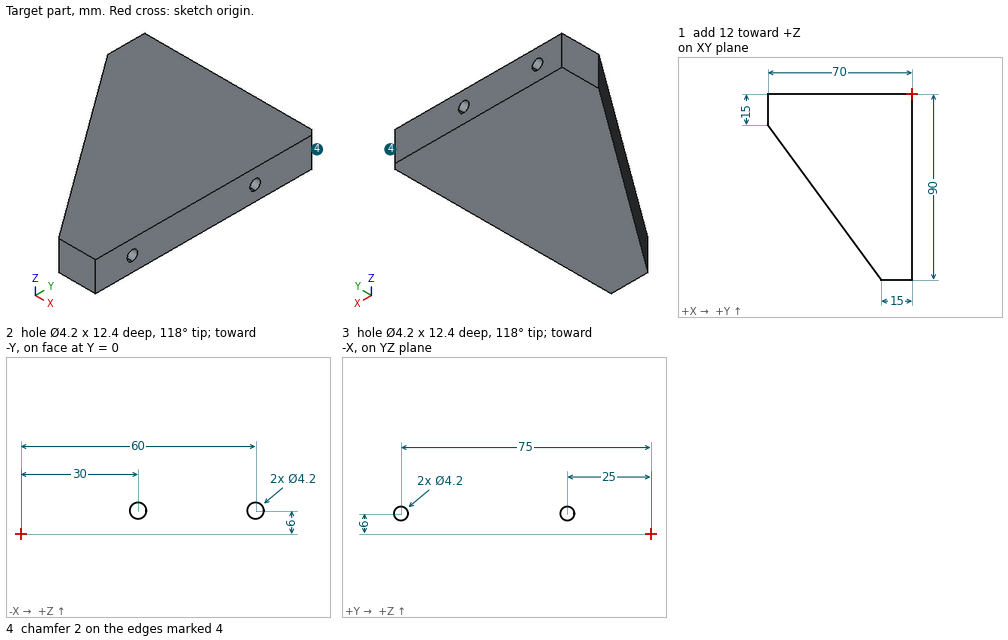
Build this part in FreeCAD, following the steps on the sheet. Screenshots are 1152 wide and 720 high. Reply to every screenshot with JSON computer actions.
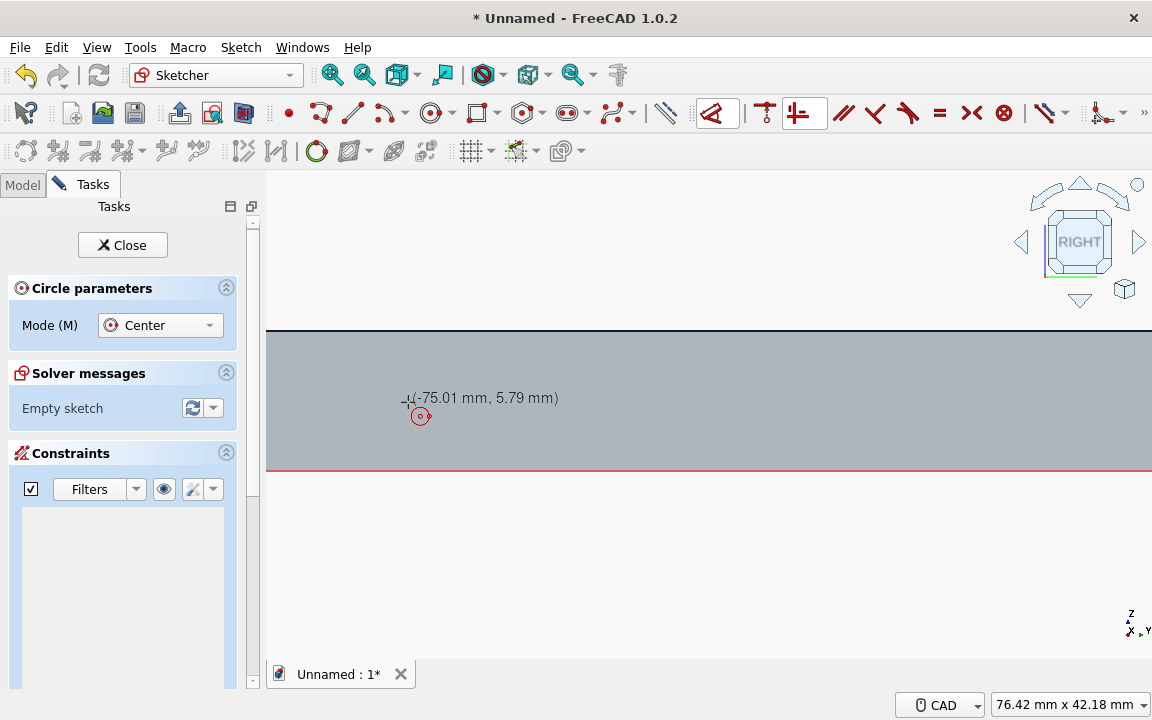
{"action": "left_click", "coordinate": [408, 401]}
{"action": "left_click", "coordinate": [425, 384]}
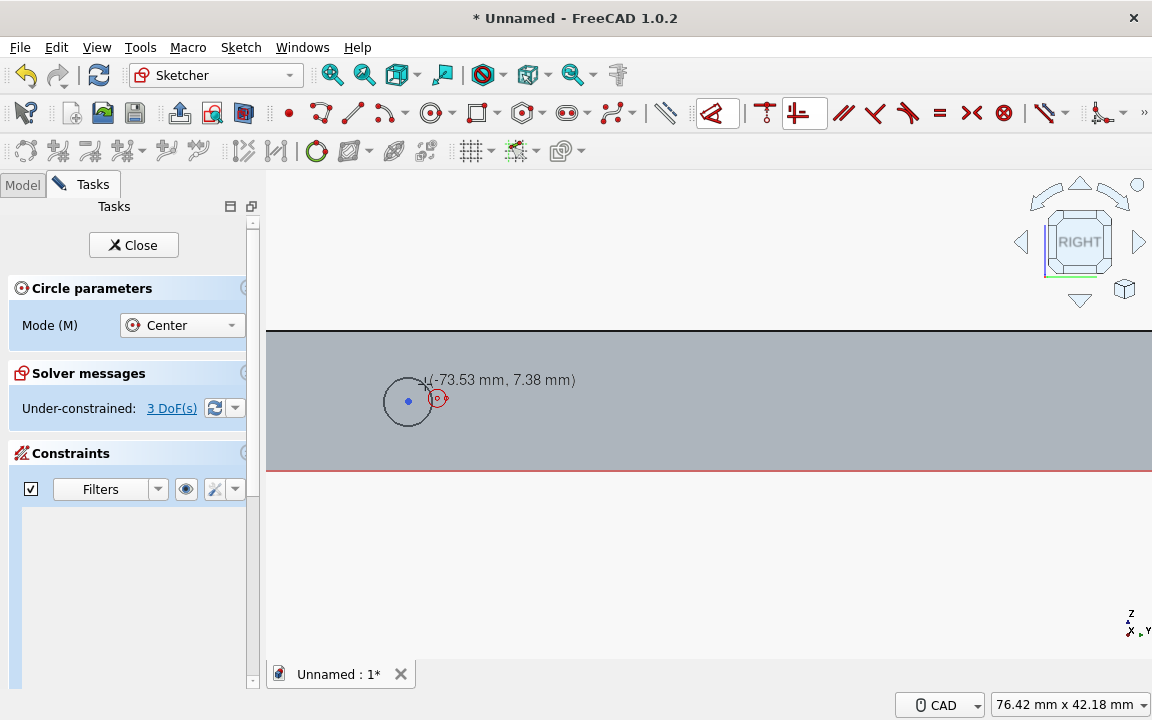
{"action": "scroll", "coordinate": [409, 403], "scroll_direction": "down", "scroll_amount": 3}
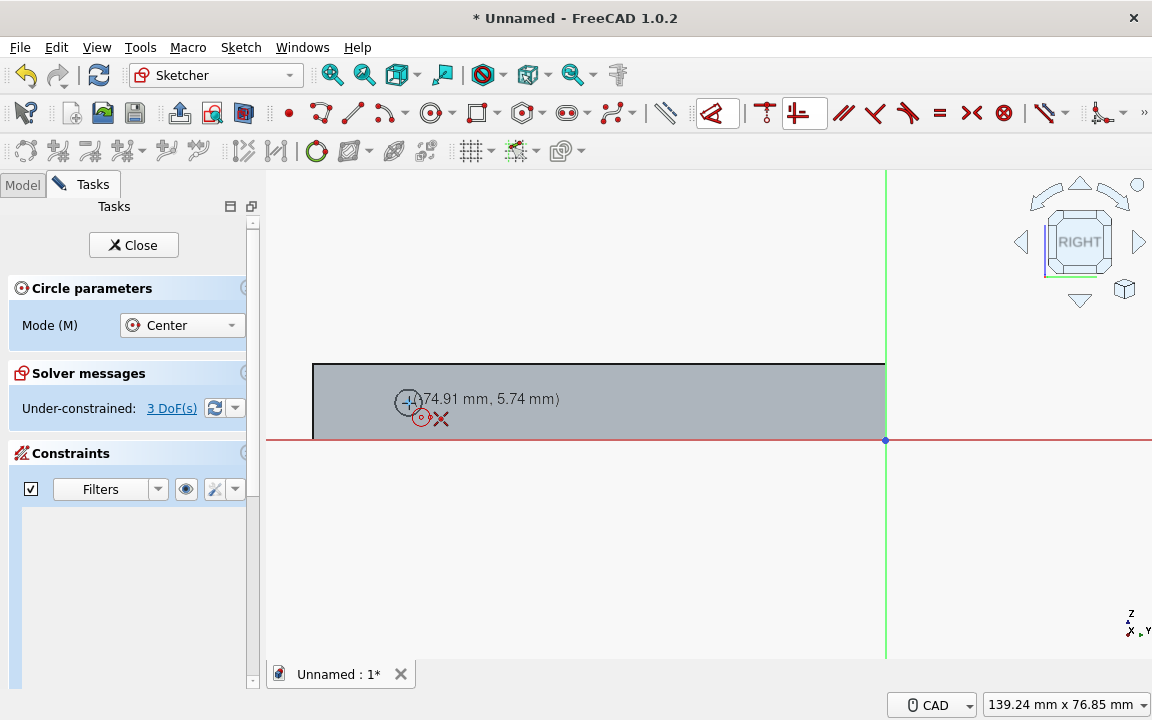
{"action": "scroll", "coordinate": [727, 402], "scroll_direction": "up", "scroll_amount": 3}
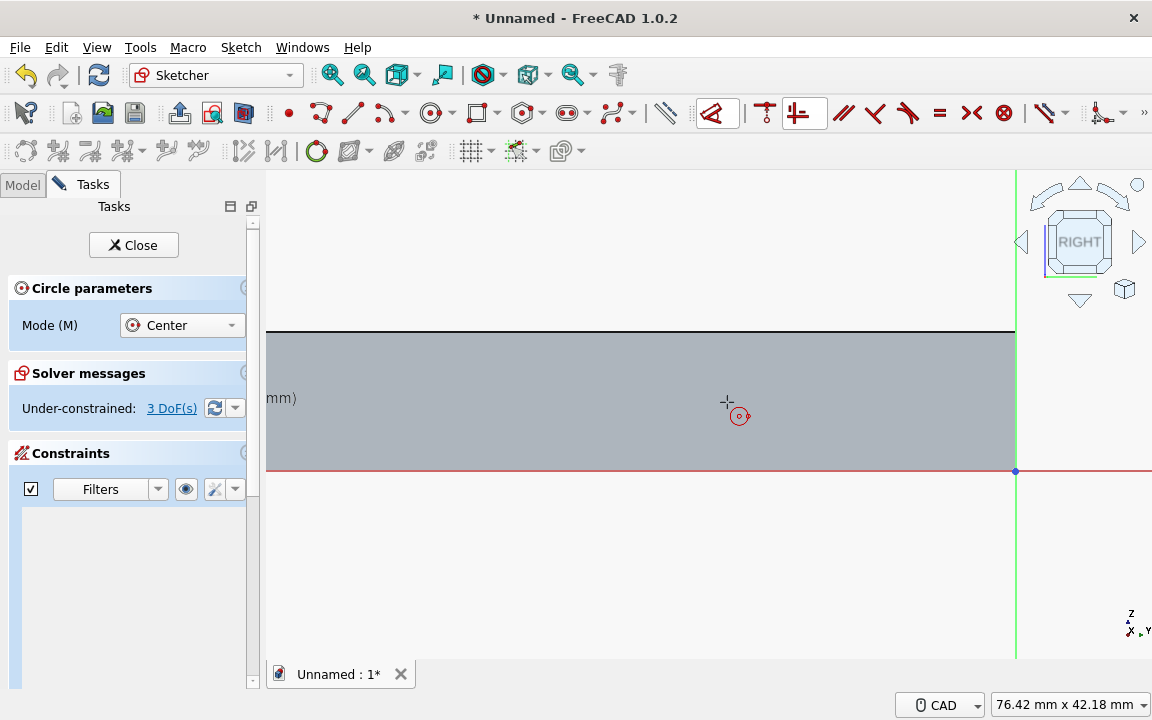
{"action": "left_click", "coordinate": [726, 402]}
{"action": "left_click", "coordinate": [743, 385]}
{"action": "key", "text": "Escape"}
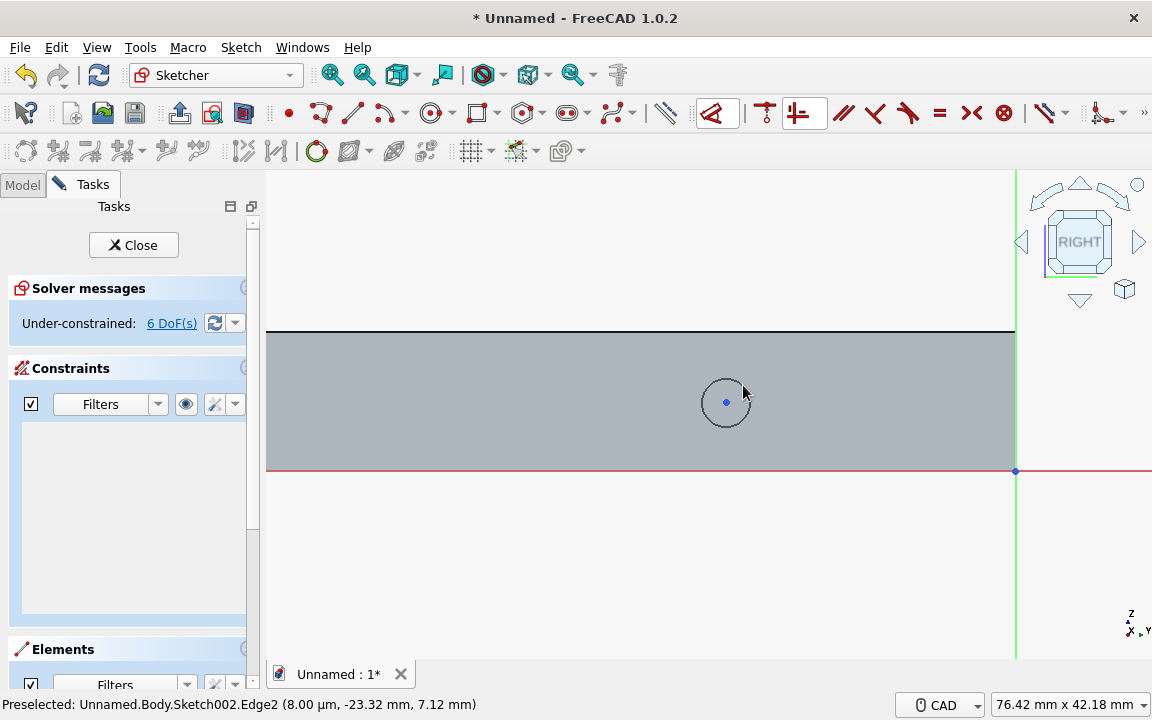
{"action": "scroll", "coordinate": [728, 402], "scroll_direction": "down", "scroll_amount": 3}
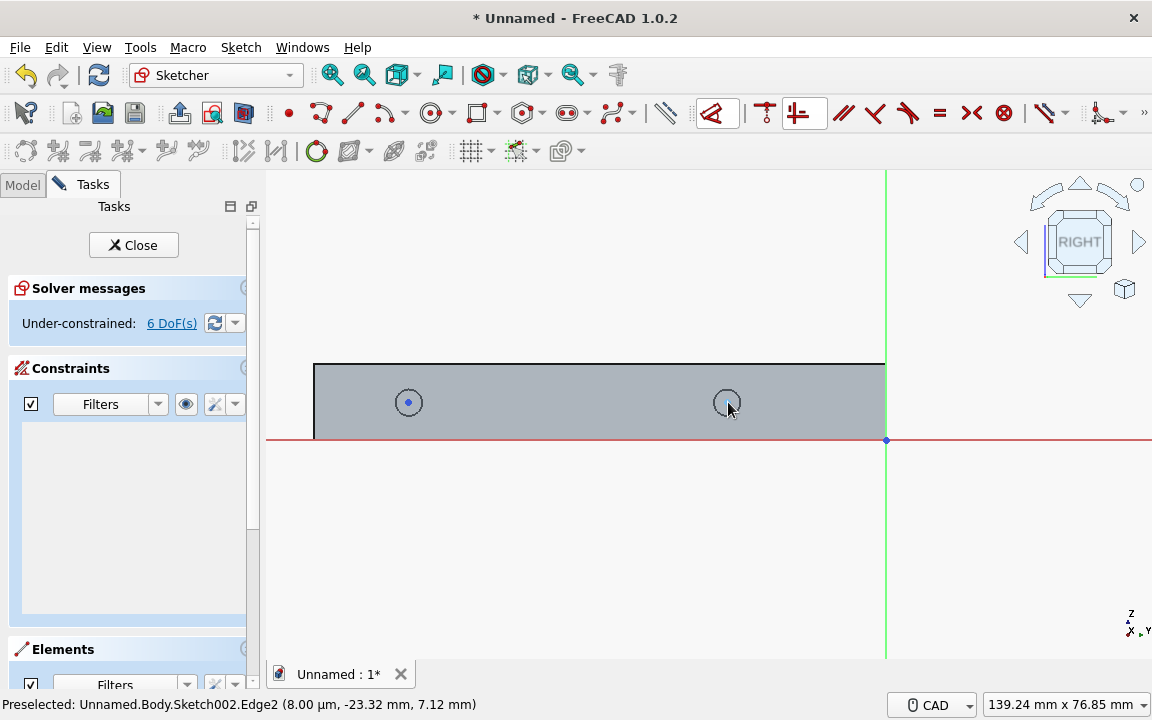
{"action": "left_click", "coordinate": [418, 393]}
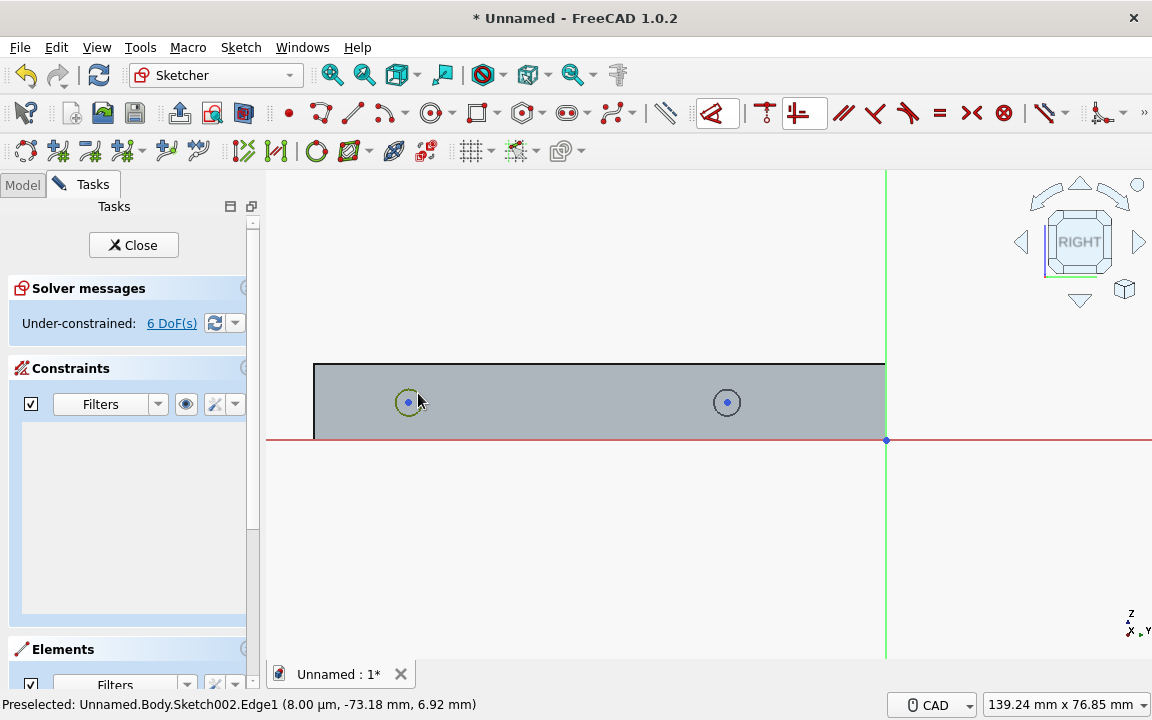
{"action": "left_click", "coordinate": [736, 393]}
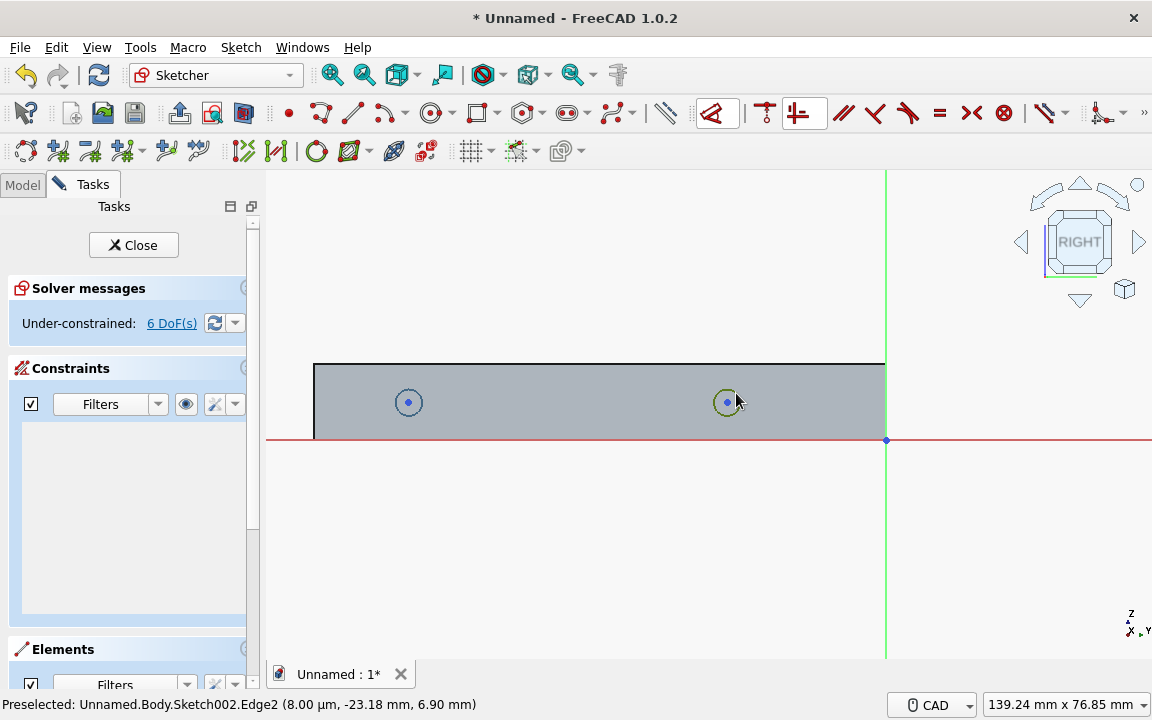
{"action": "left_click", "coordinate": [940, 114]}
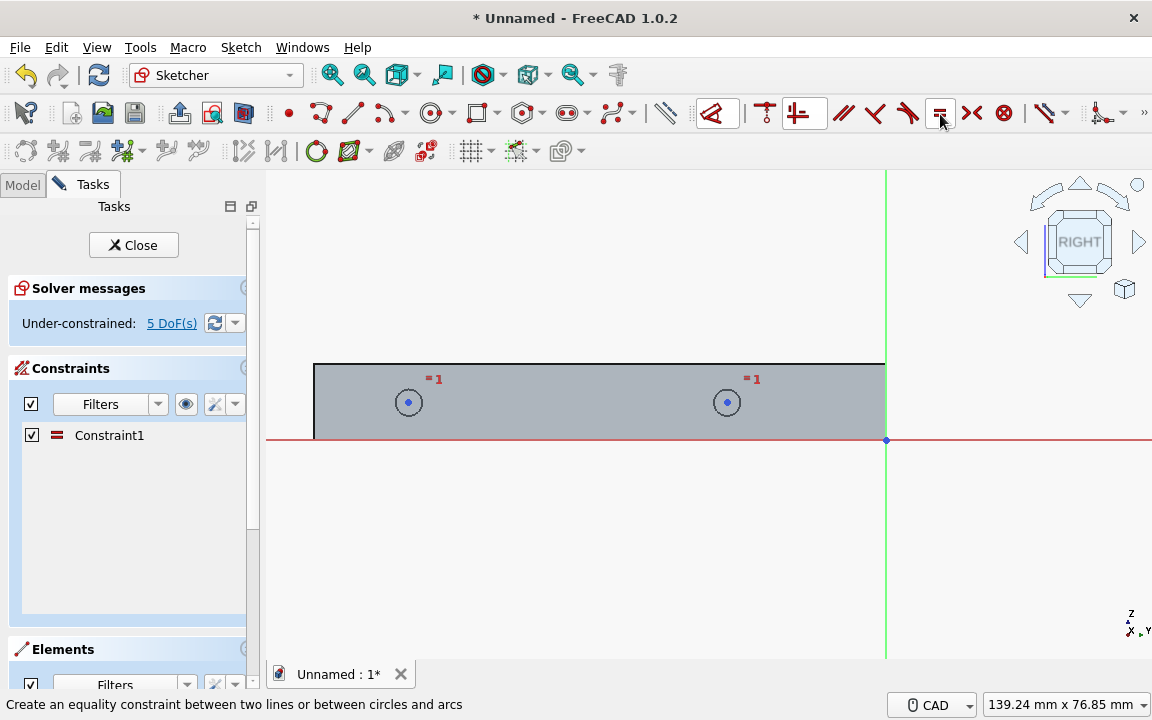
{"action": "left_click", "coordinate": [409, 403]}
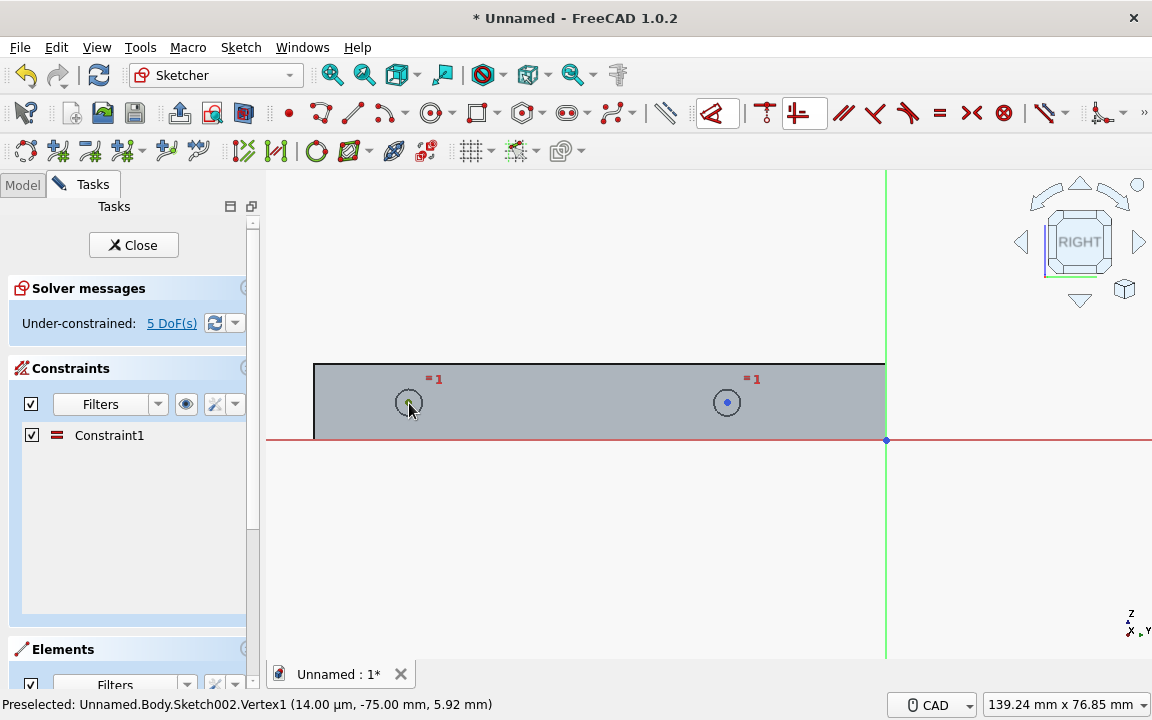
{"action": "left_click", "coordinate": [727, 403]}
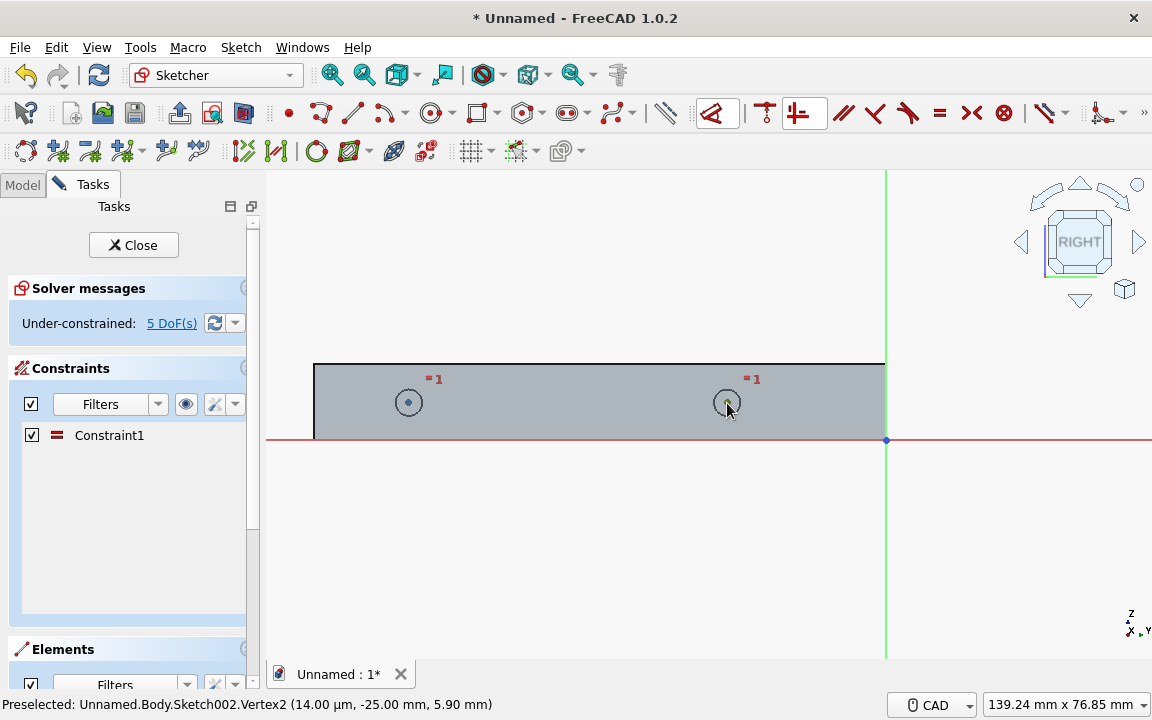
{"action": "key", "text": "h"}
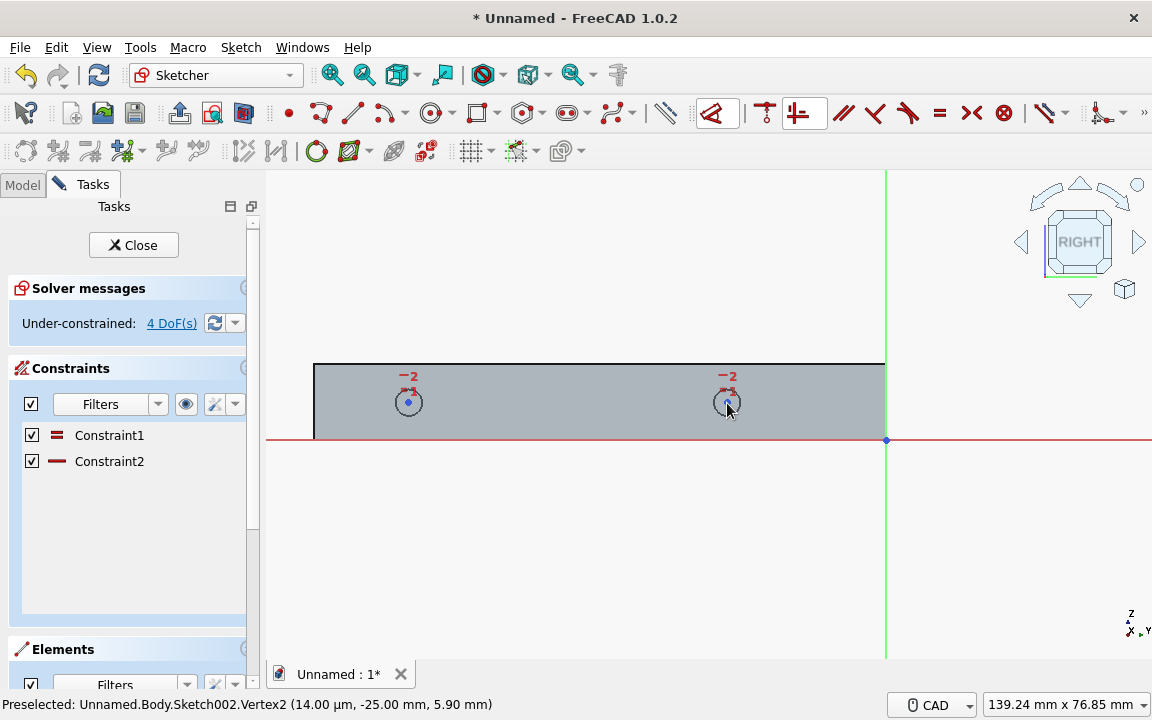
{"action": "scroll", "coordinate": [418, 393], "scroll_direction": "up", "scroll_amount": 2}